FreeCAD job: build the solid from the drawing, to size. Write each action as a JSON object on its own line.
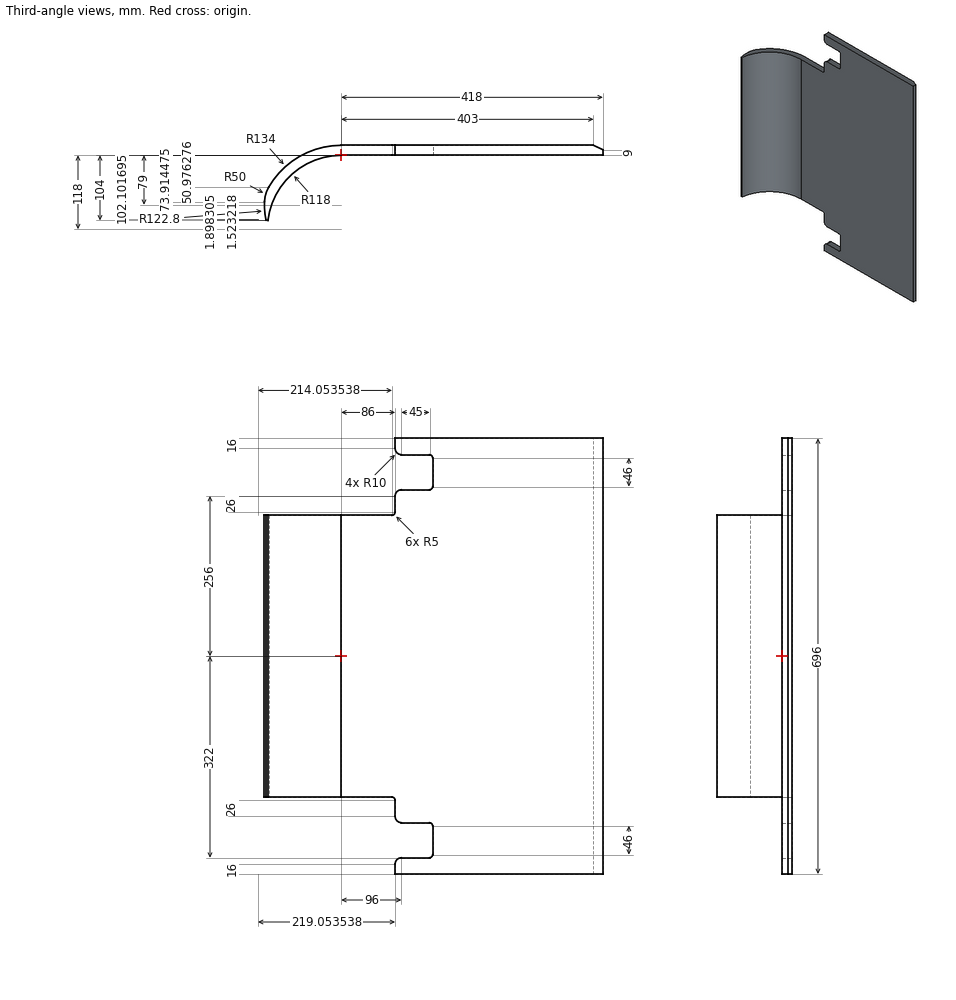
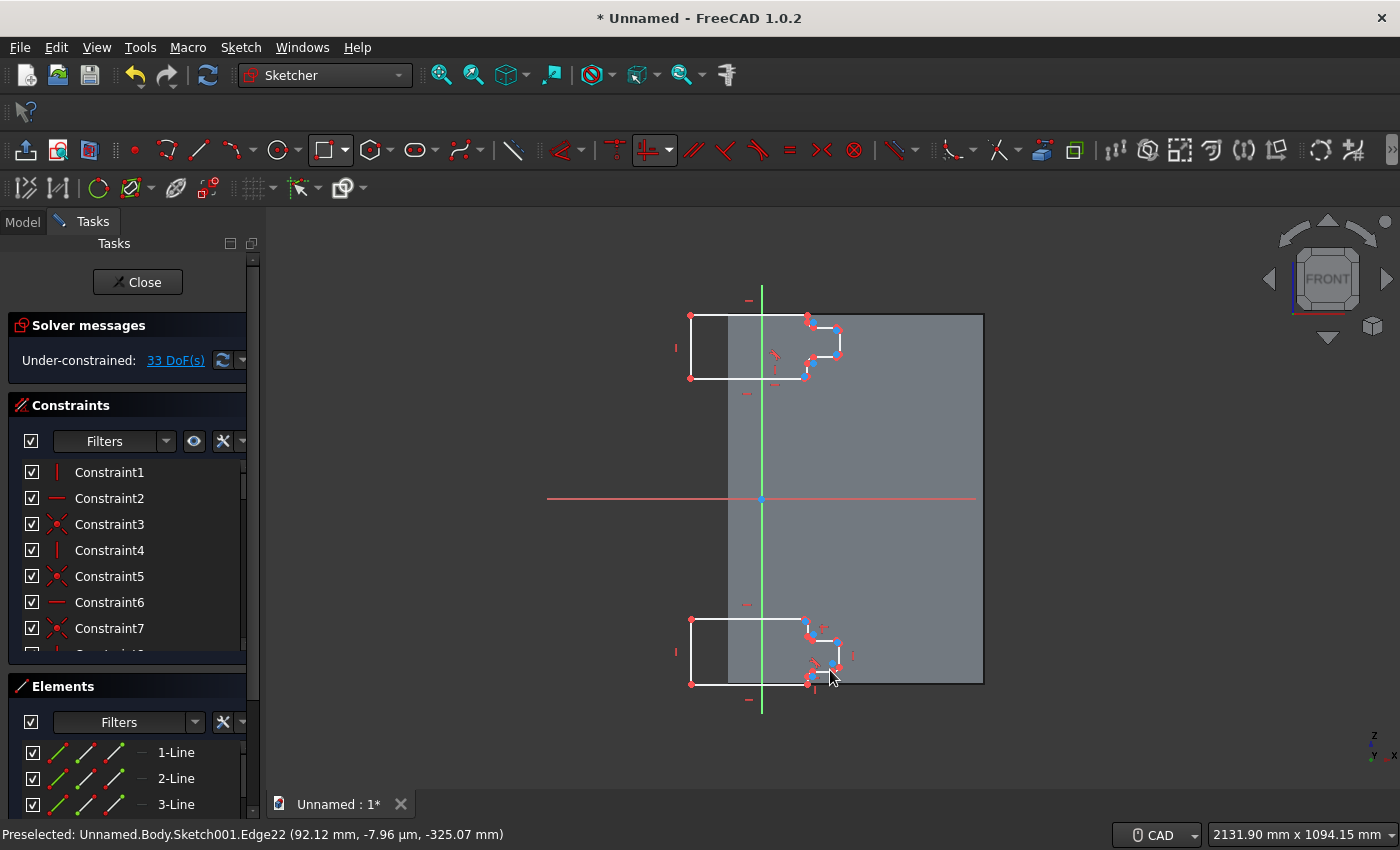
{"action": "left_click", "coordinate": [725, 619]}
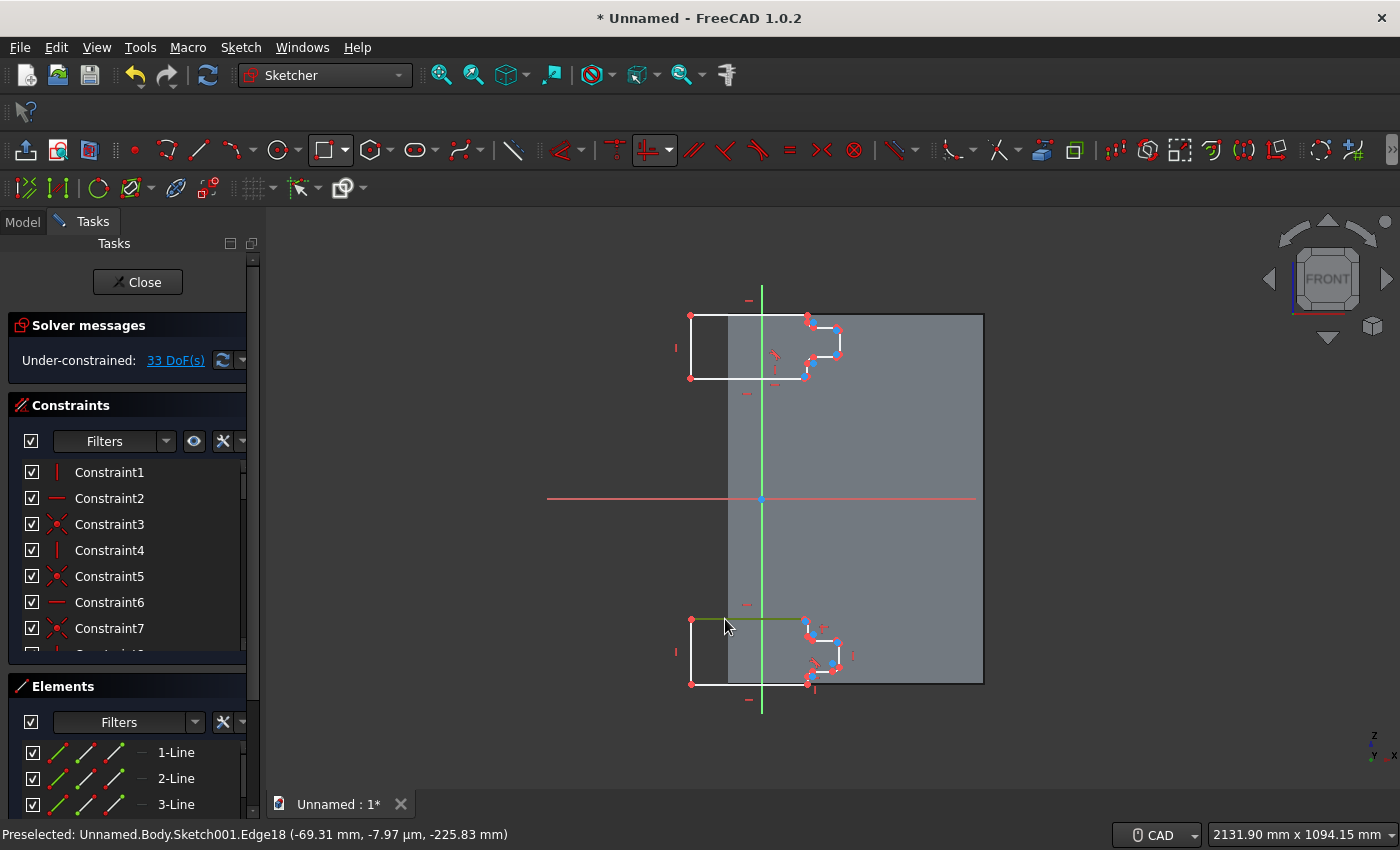
{"action": "scroll", "coordinate": [807, 620], "scroll_direction": "up", "scroll_amount": 10}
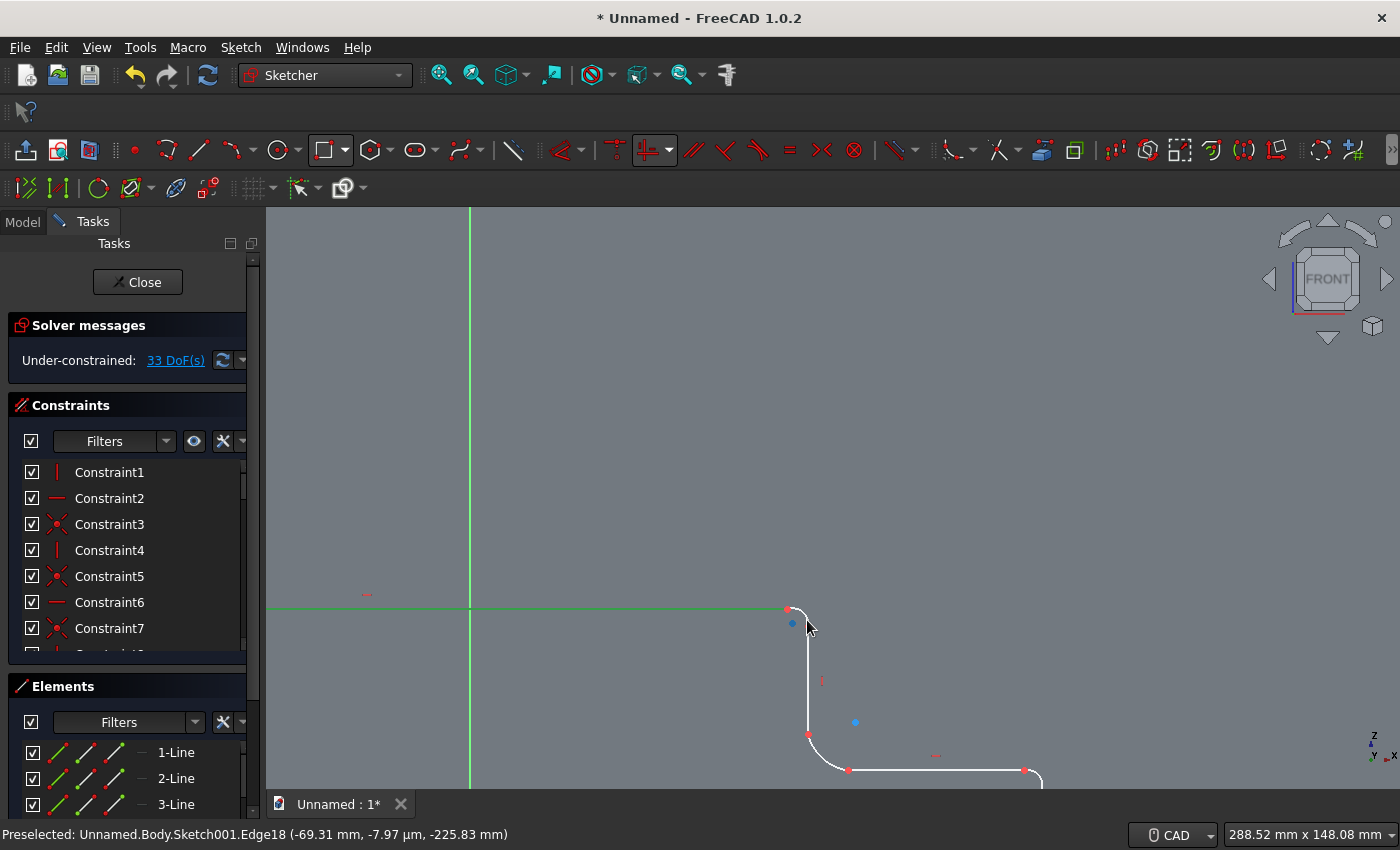
{"action": "left_click", "coordinate": [803, 612]}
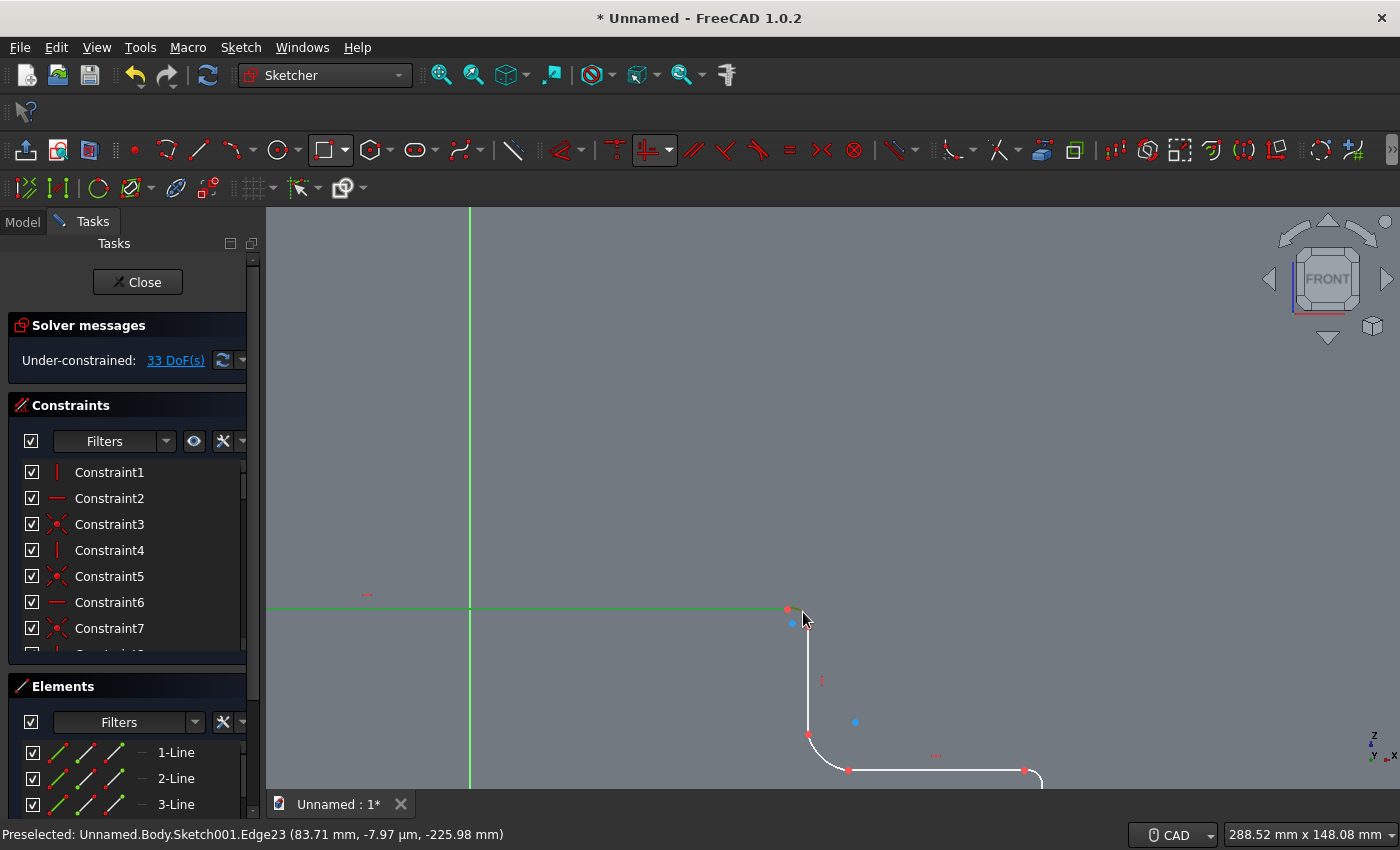
{"action": "left_click", "coordinate": [758, 150]}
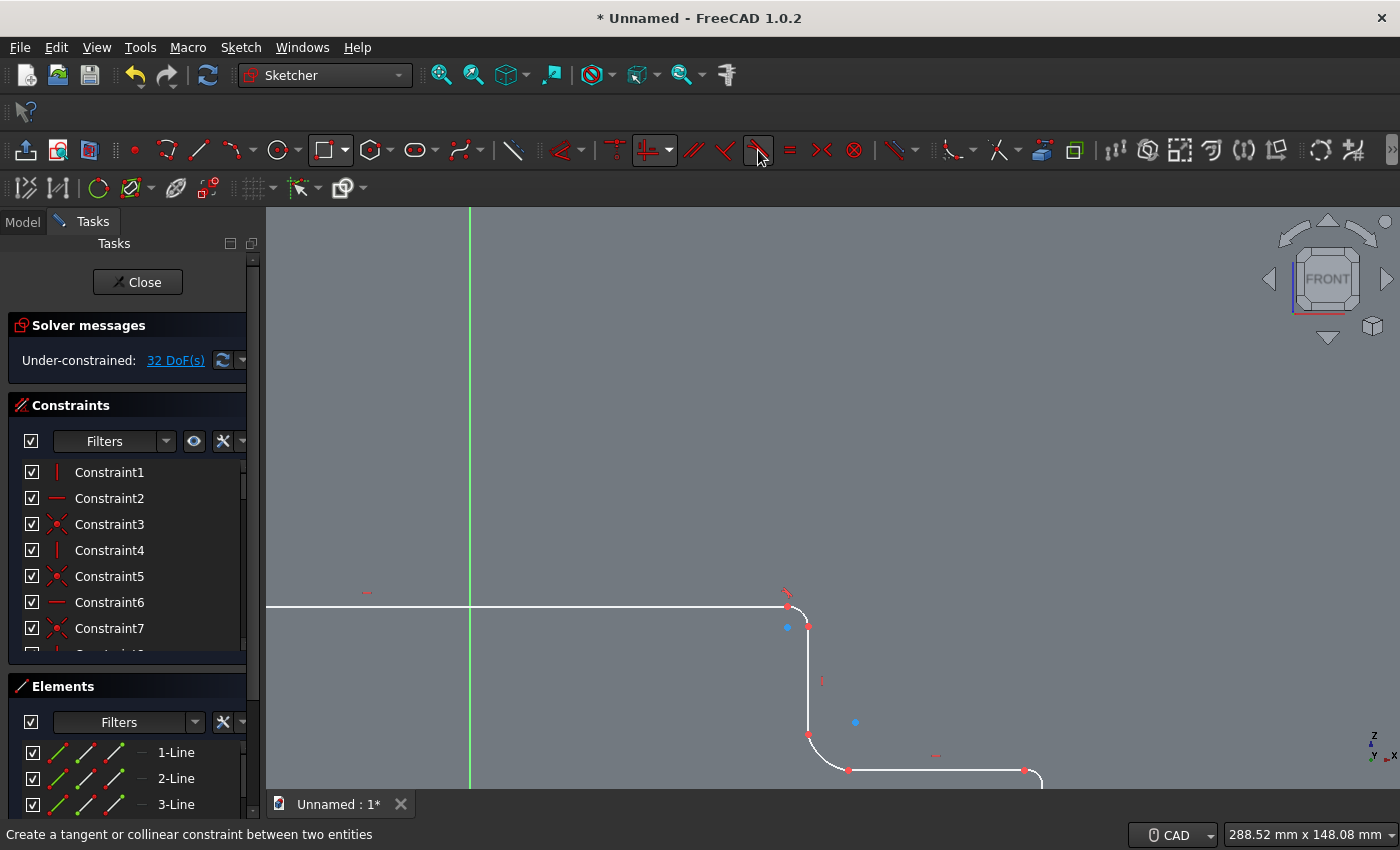
{"action": "left_click", "coordinate": [808, 659]}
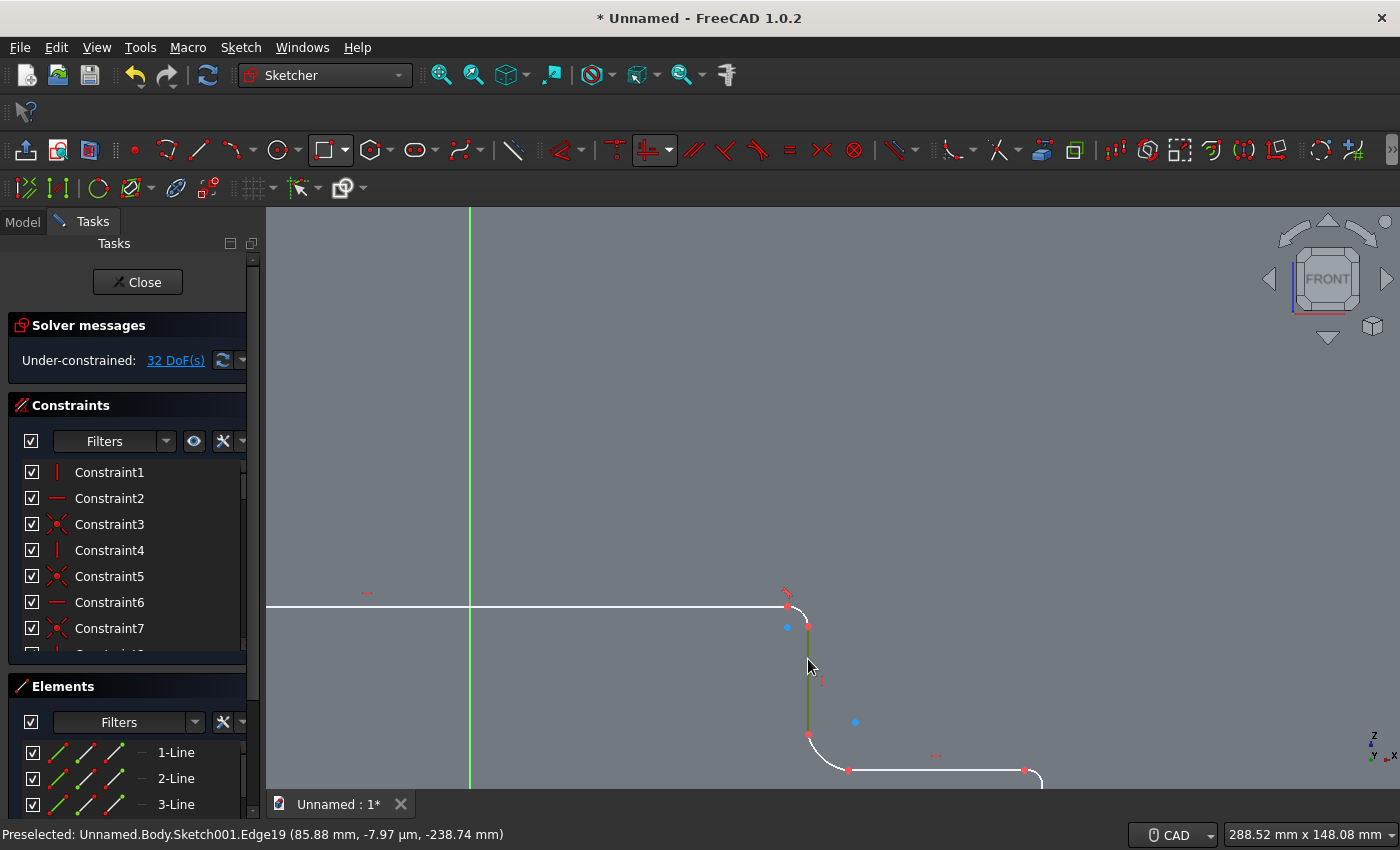
{"action": "scroll", "coordinate": [806, 618], "scroll_direction": "up", "scroll_amount": 2}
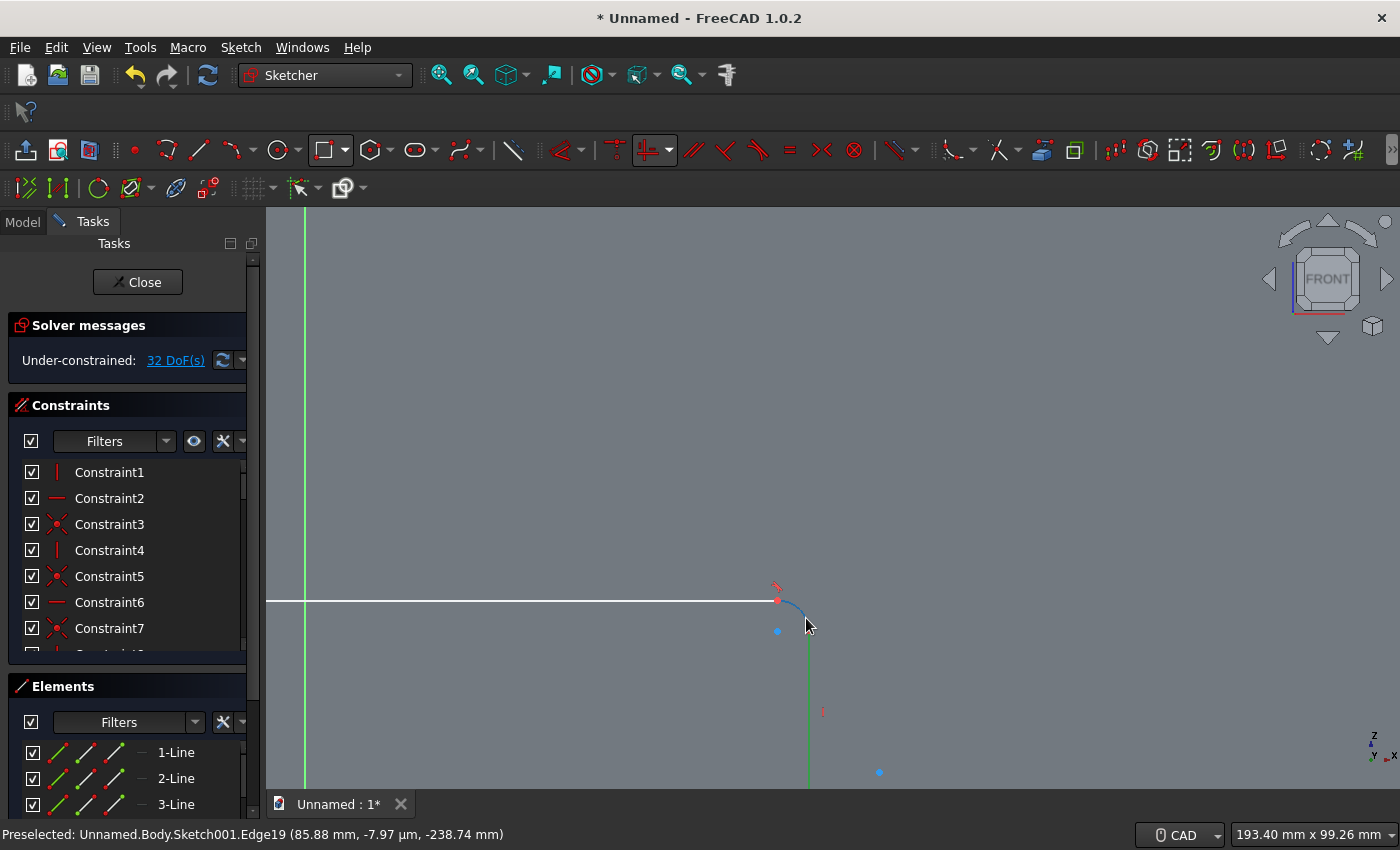
{"action": "left_click", "coordinate": [805, 617]}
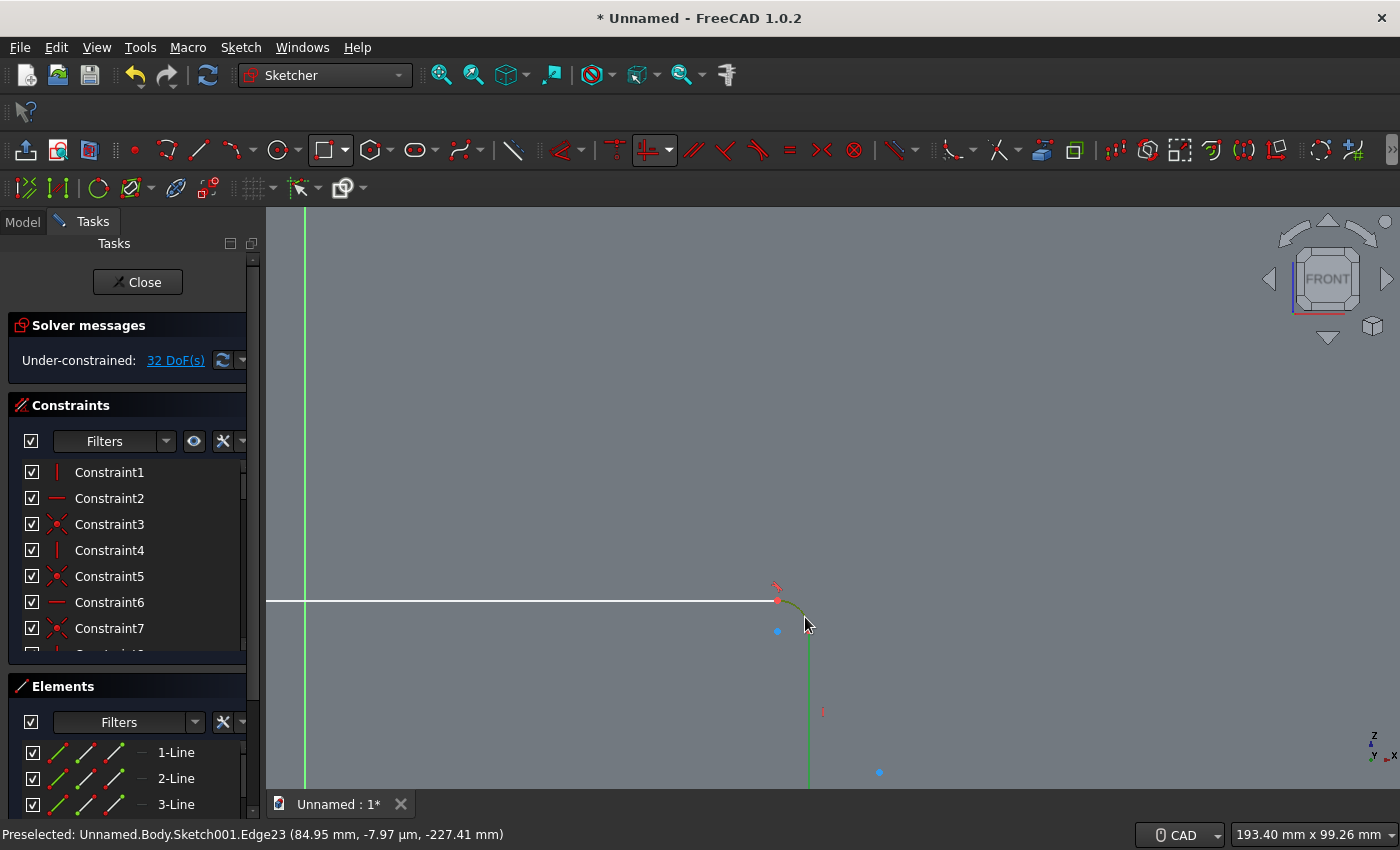
{"action": "left_click", "coordinate": [758, 150]}